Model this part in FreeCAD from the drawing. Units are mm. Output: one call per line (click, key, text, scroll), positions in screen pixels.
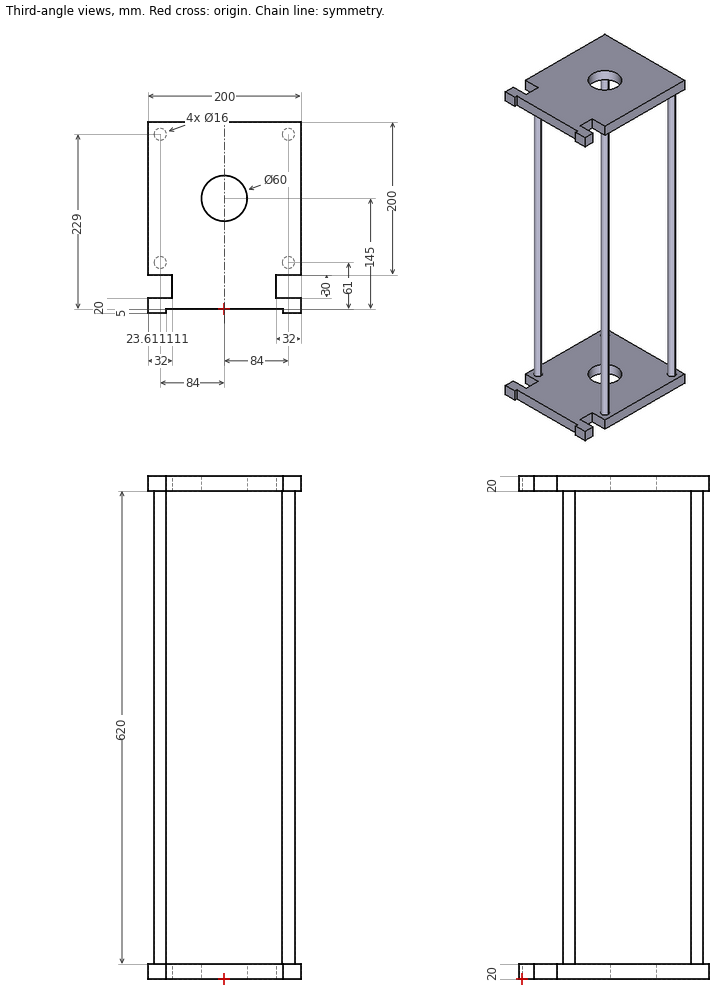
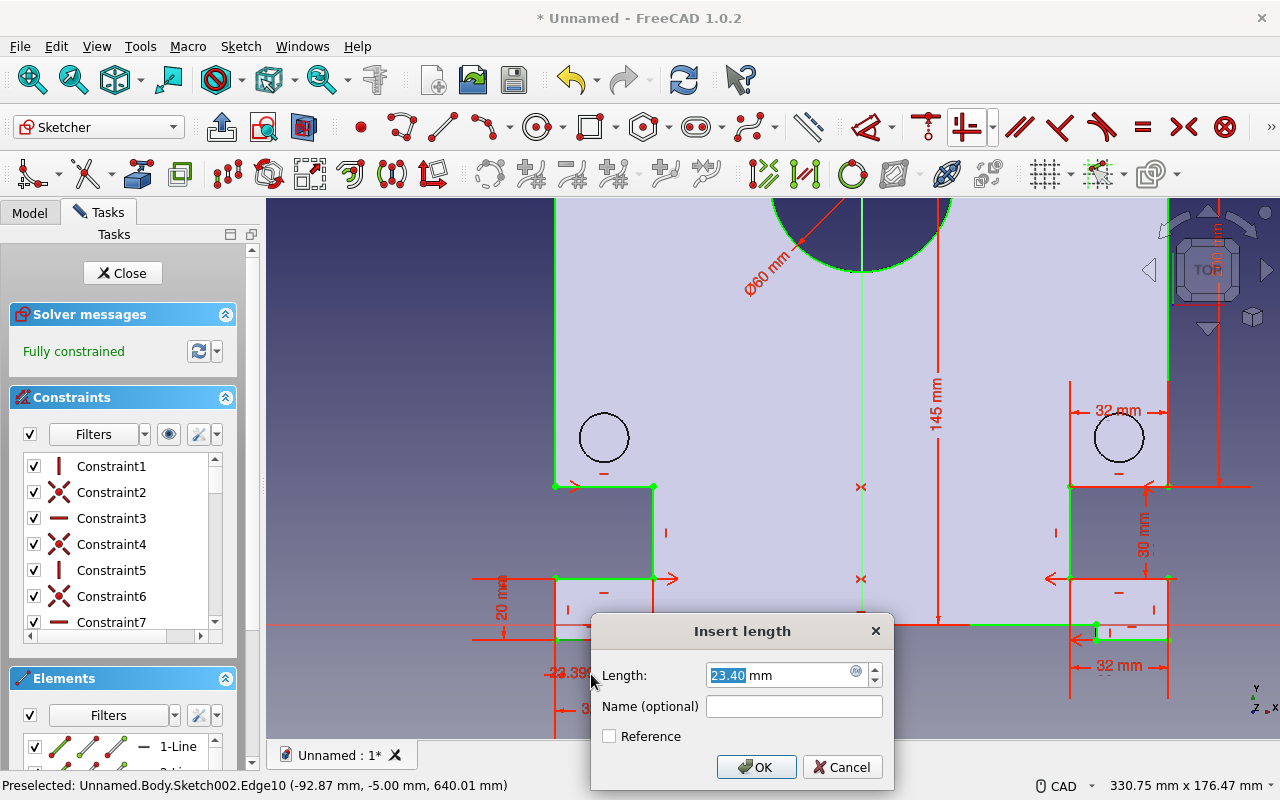
text(23.611111)
key(Return)
key(Escape)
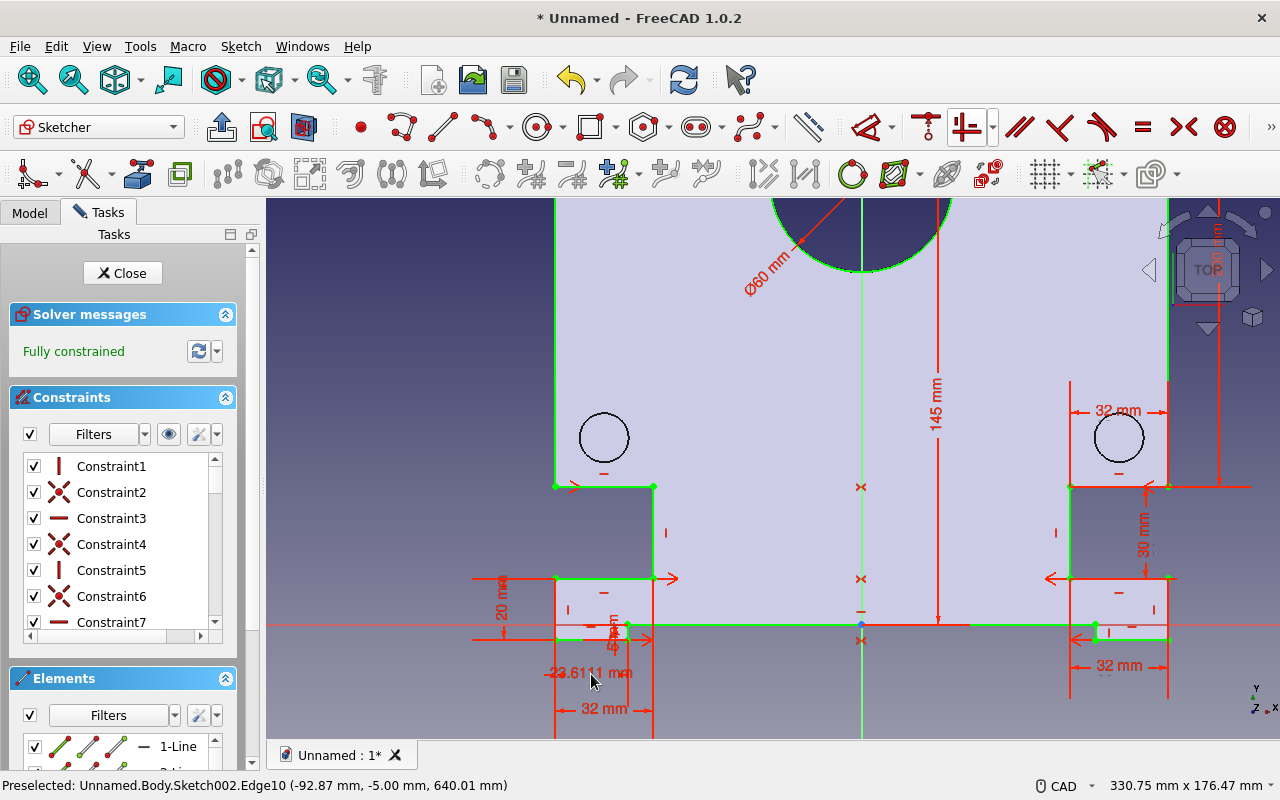
click(123, 273)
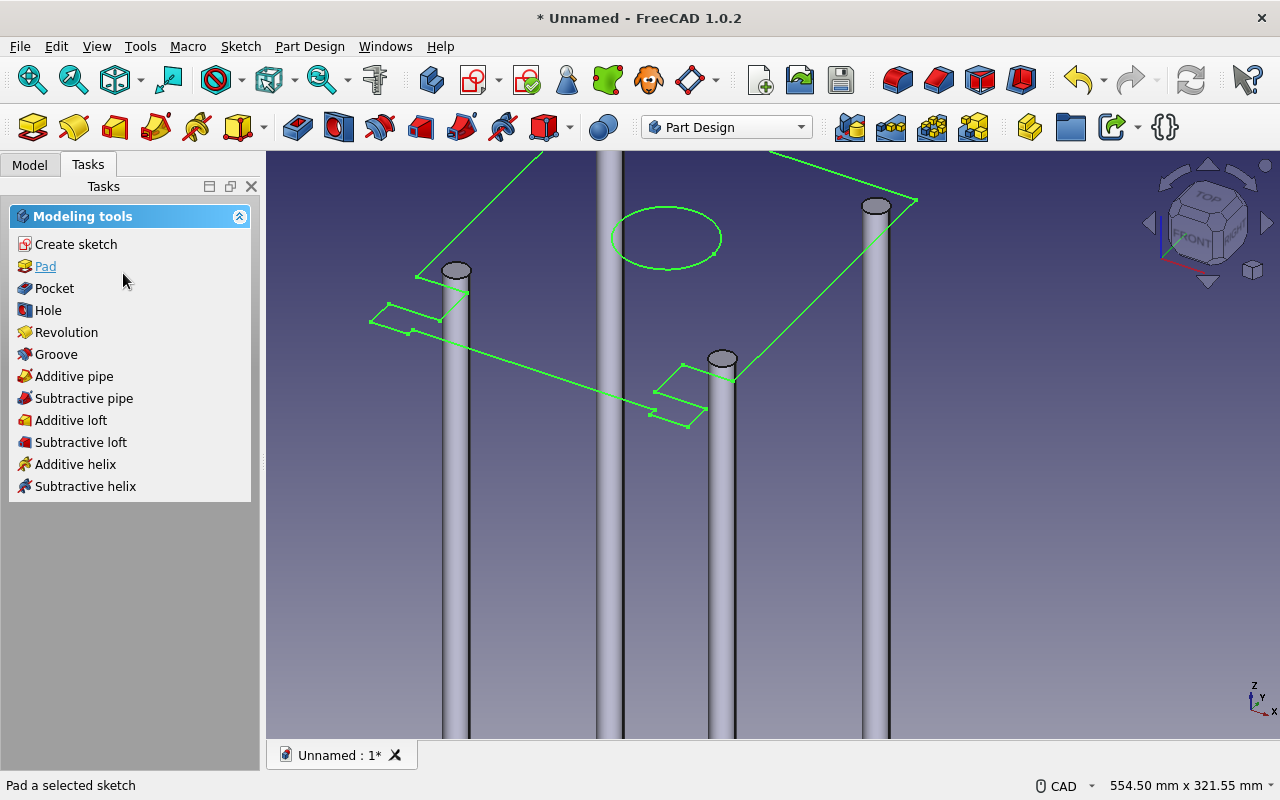
click(33, 128)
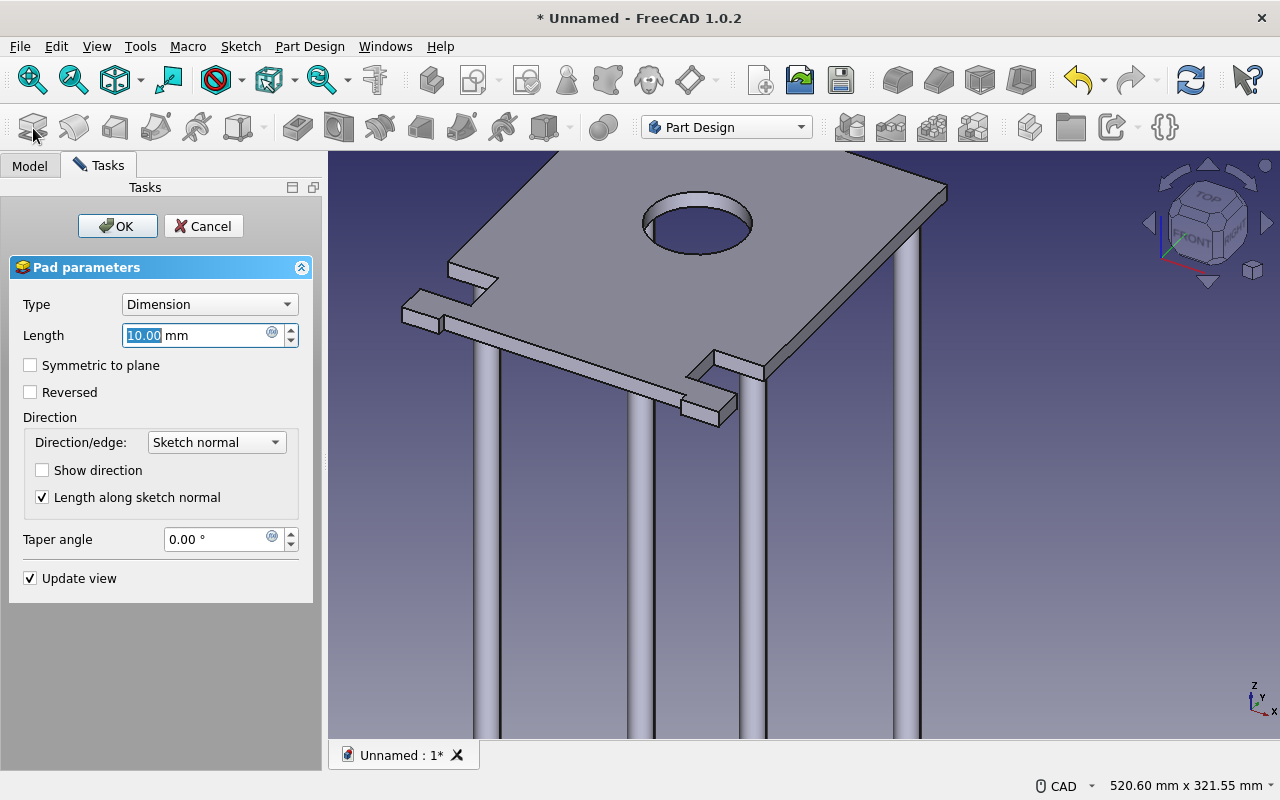
text(20)
key(Tab)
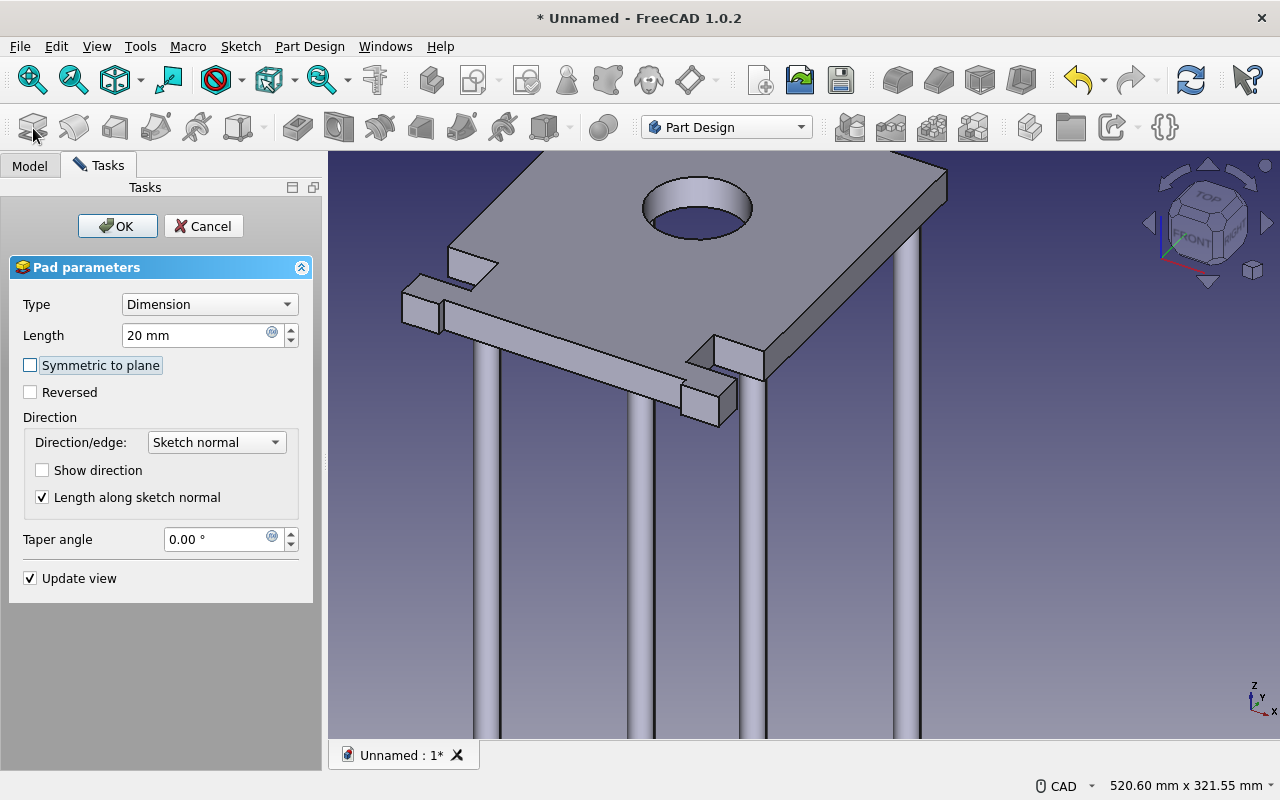
click(118, 226)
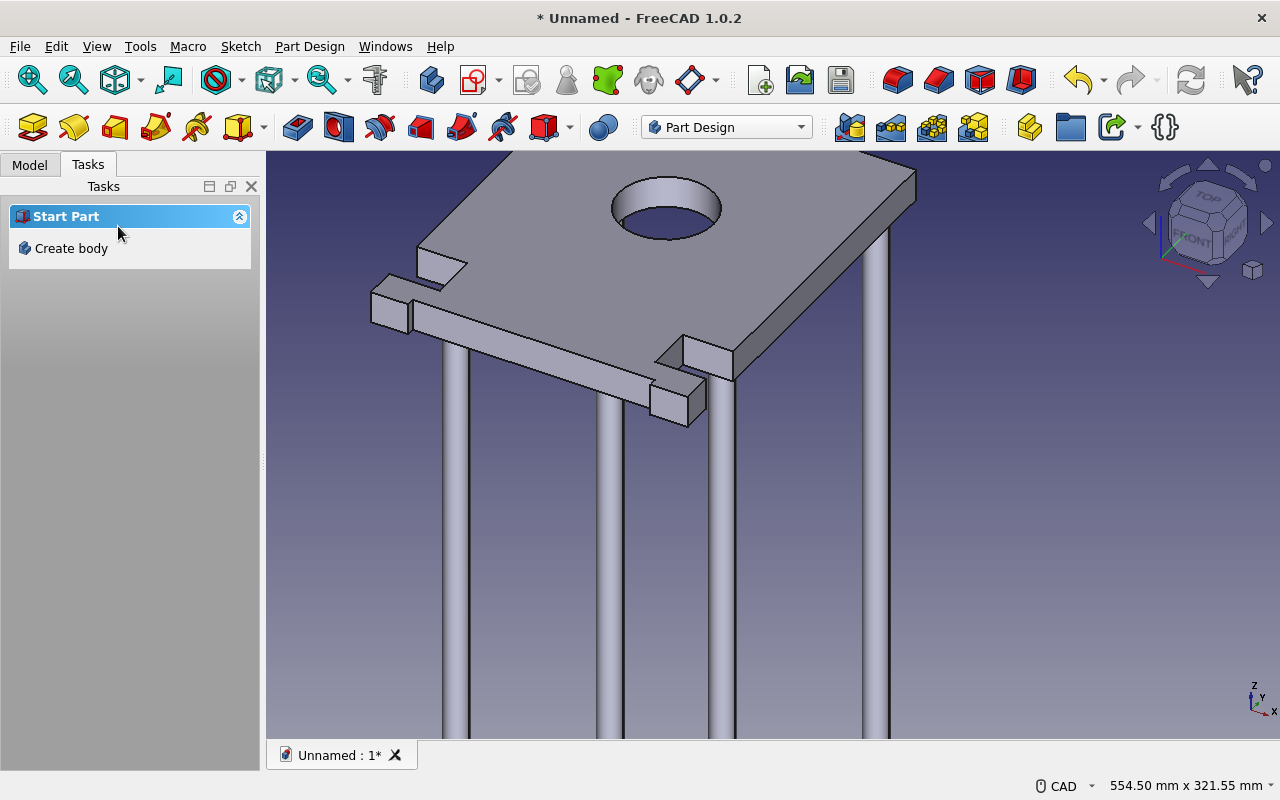
key(0)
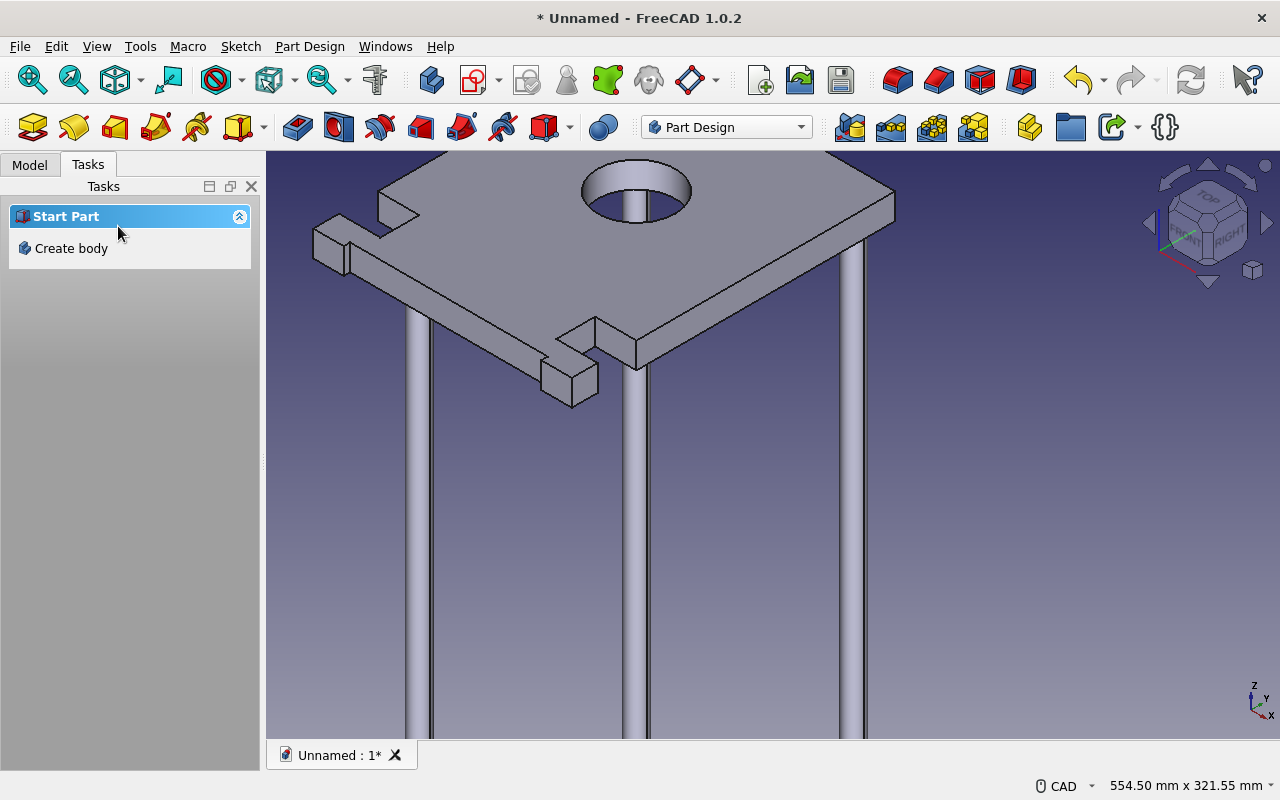
click(33, 80)